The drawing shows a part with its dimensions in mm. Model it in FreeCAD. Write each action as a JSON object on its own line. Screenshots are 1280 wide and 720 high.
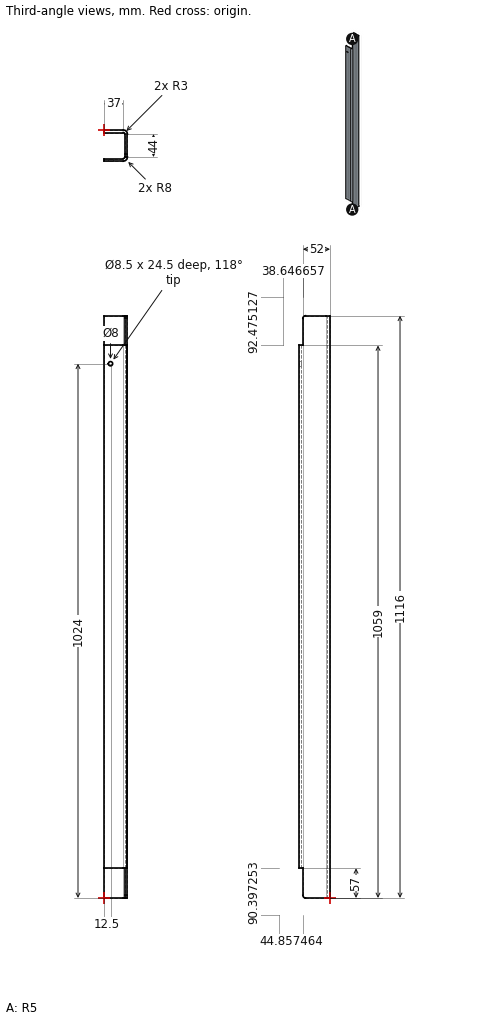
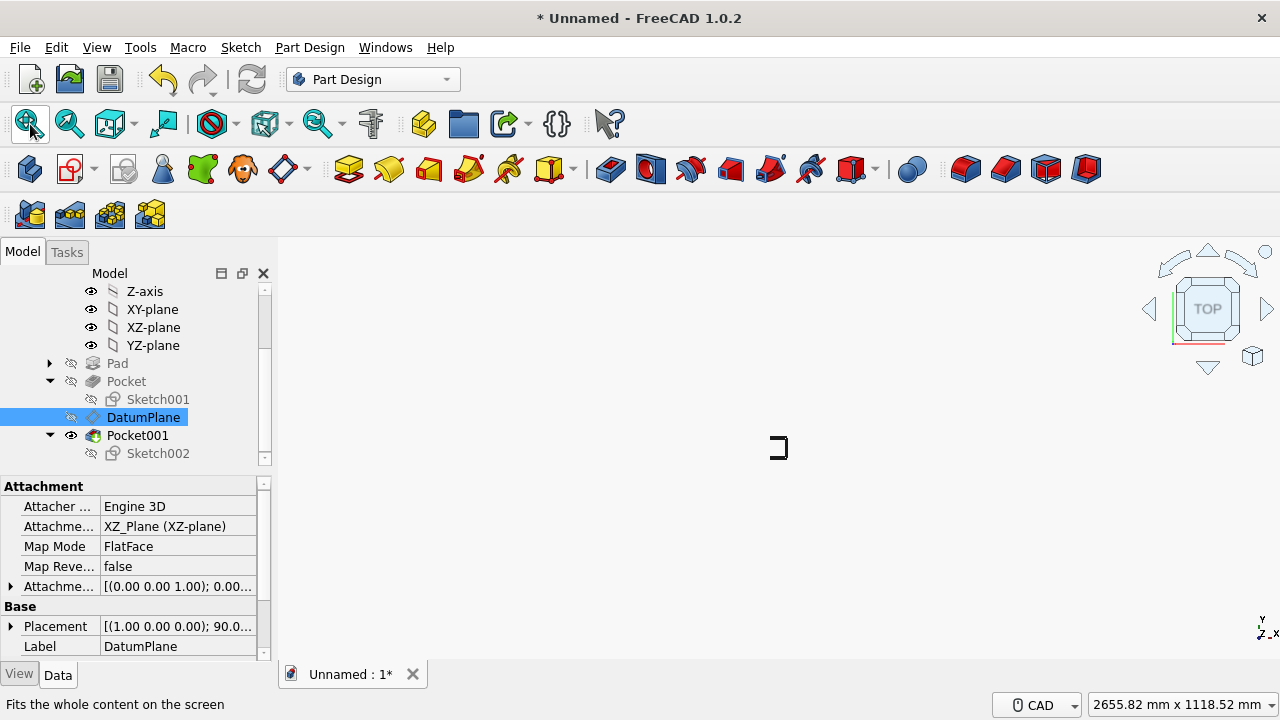
{"action": "scroll", "coordinate": [787, 455], "scroll_direction": "up", "scroll_amount": 15}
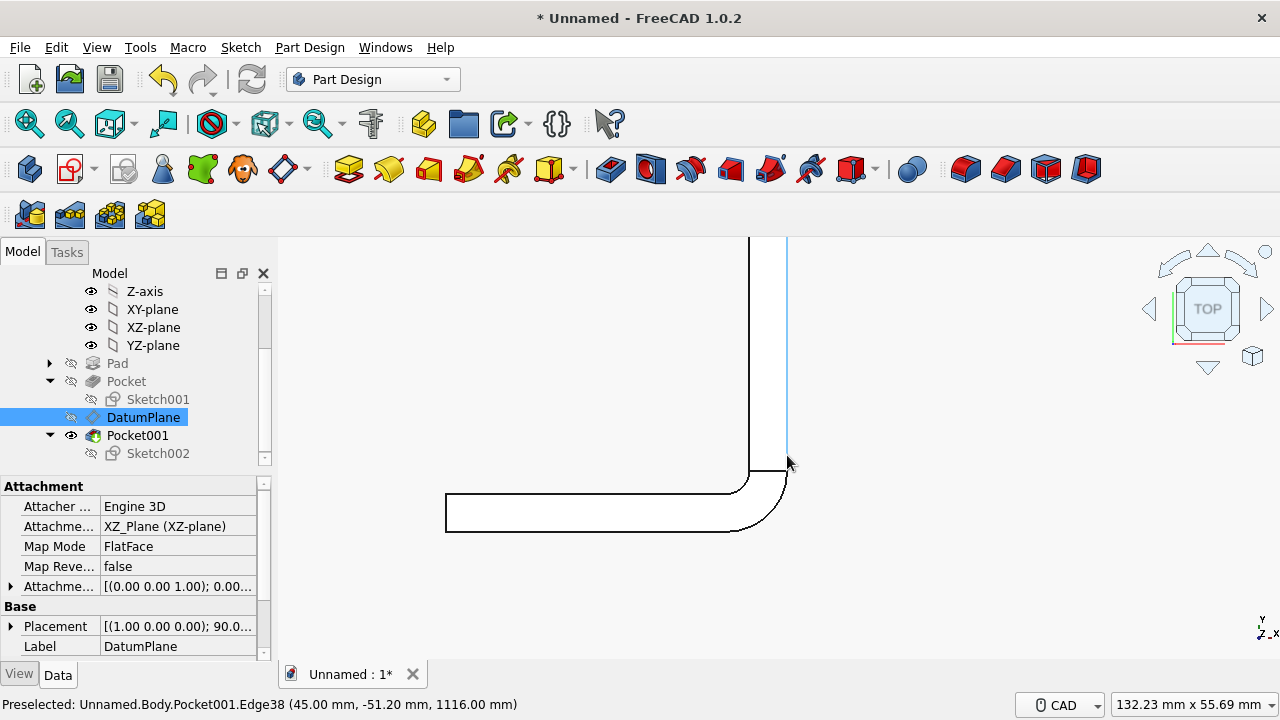
{"action": "left_click", "coordinate": [768, 470]}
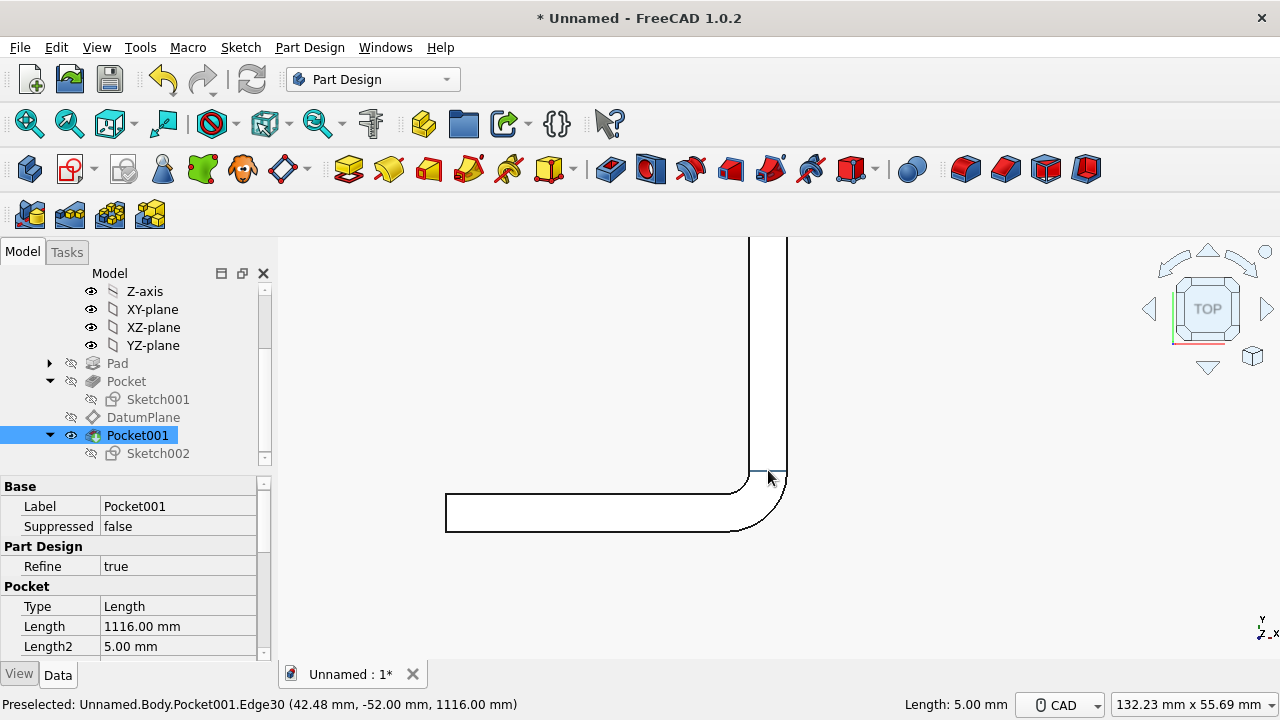
{"action": "key", "text": "v f"}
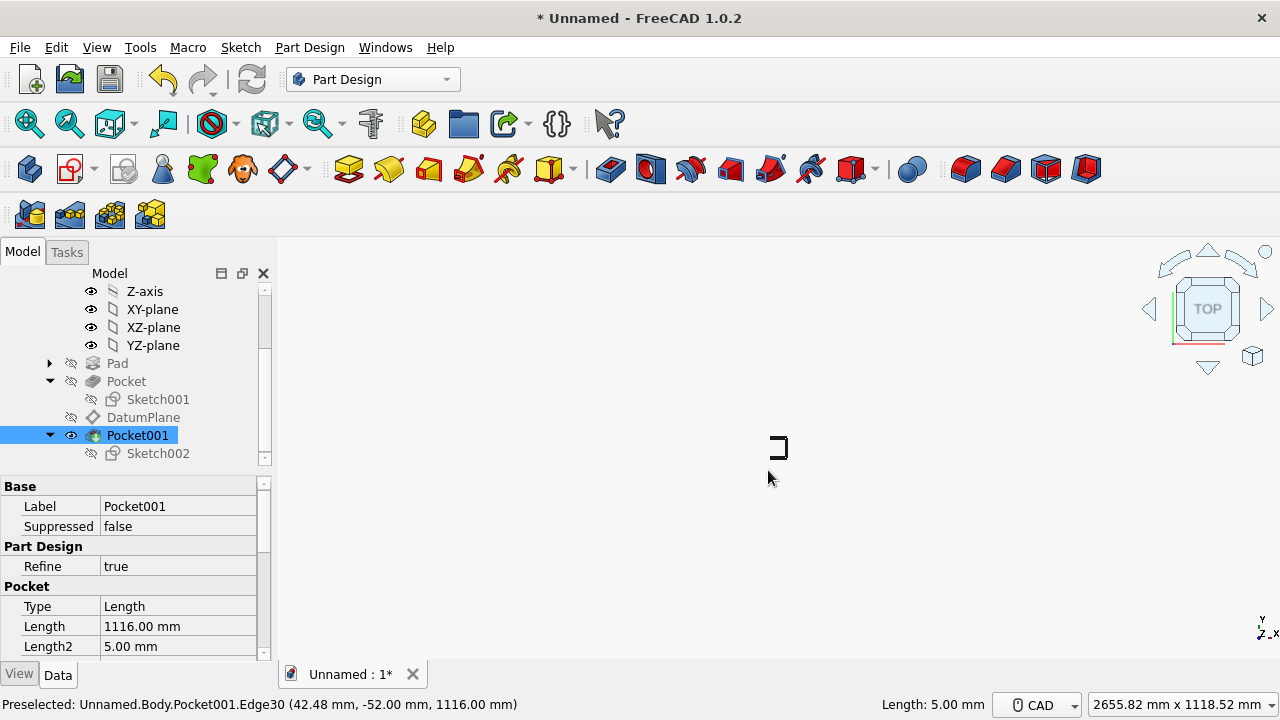
{"action": "key", "text": "1"}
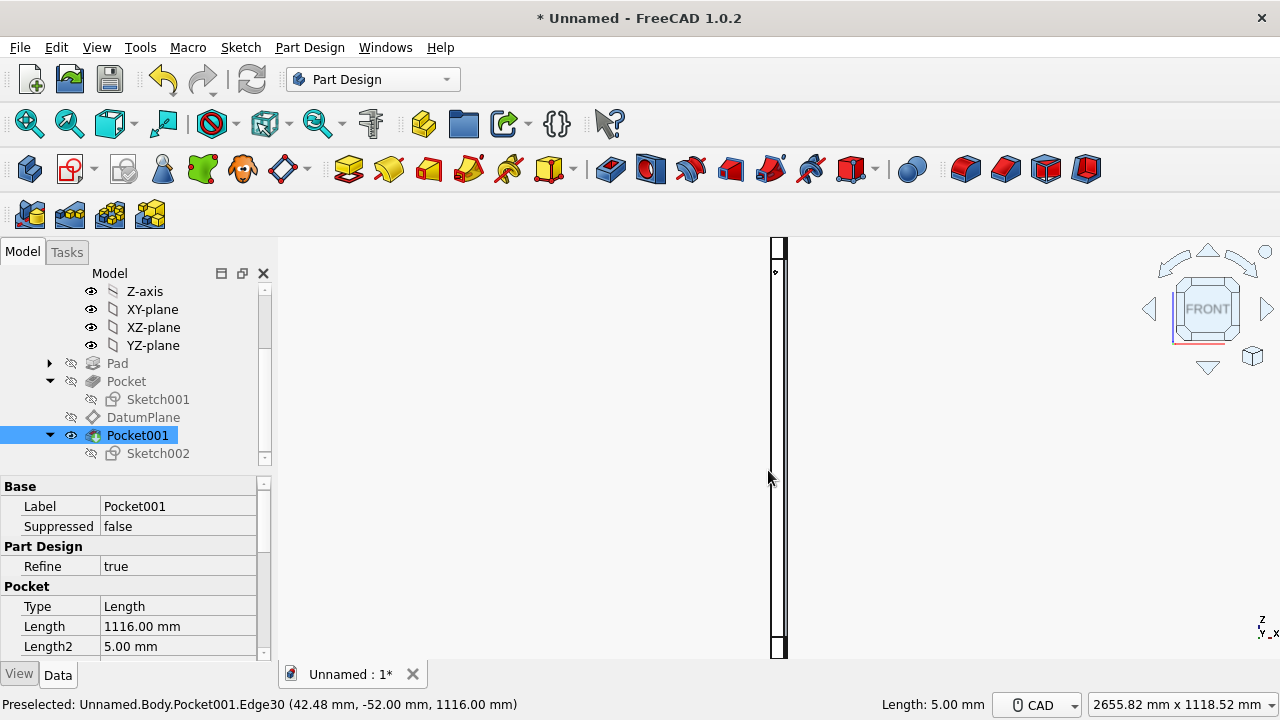
{"action": "left_click", "coordinate": [30, 124]}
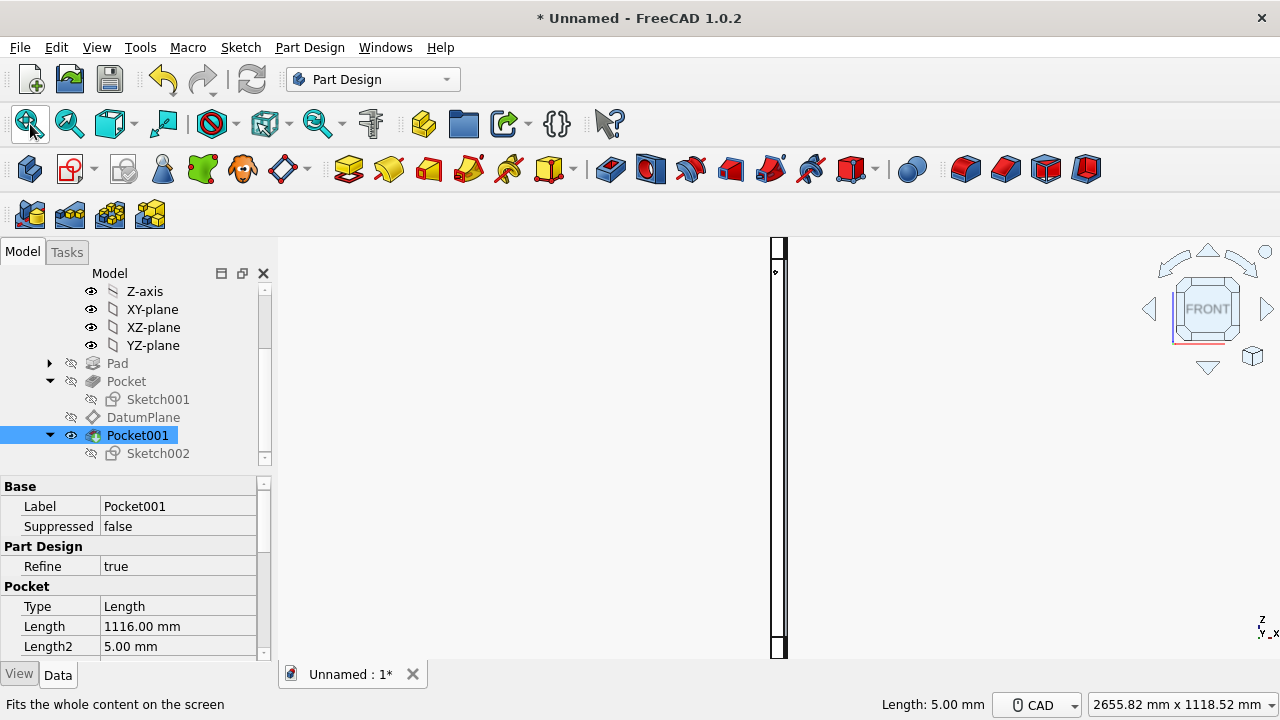
{"action": "key", "text": "3"}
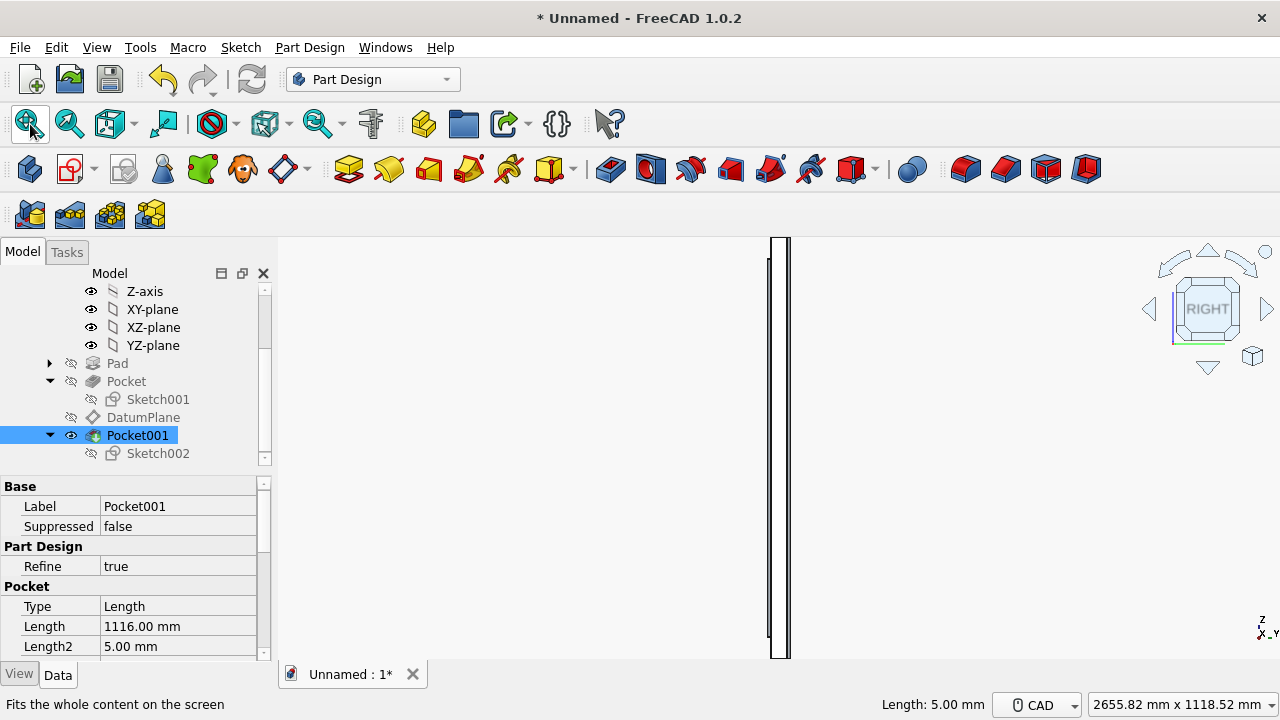
{"action": "key", "text": "v f"}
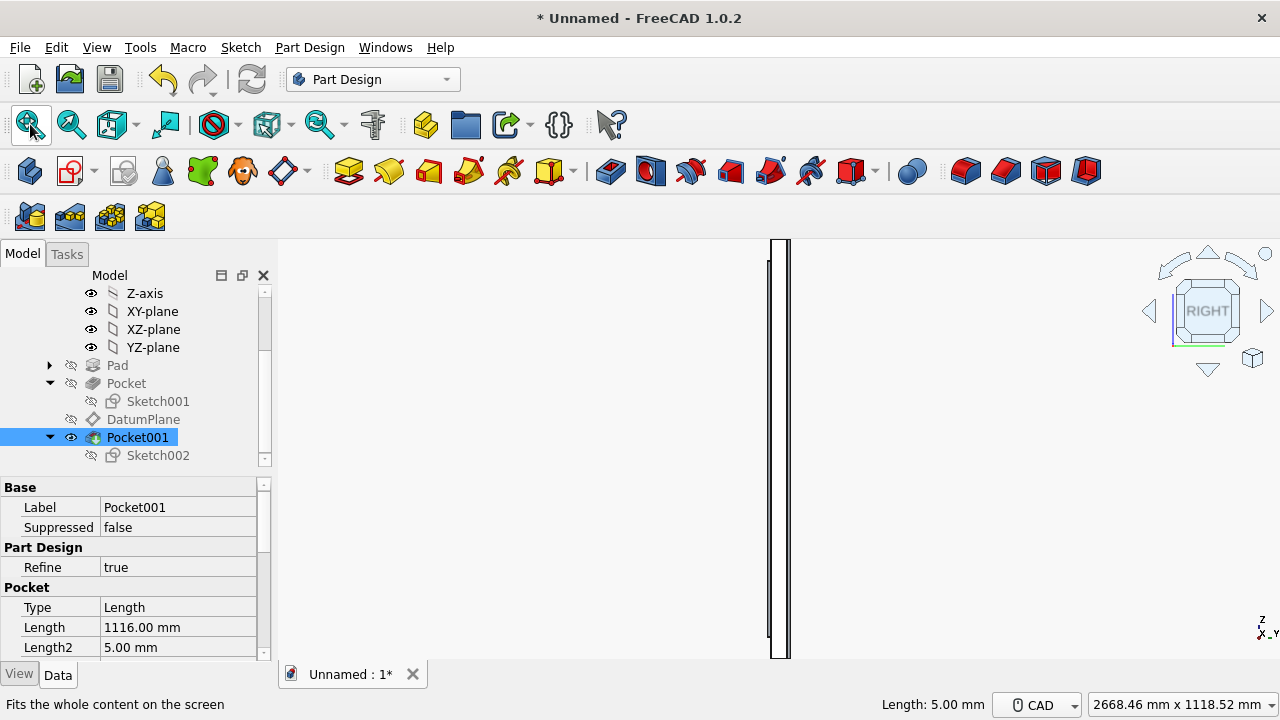
{"action": "key", "text": "5"}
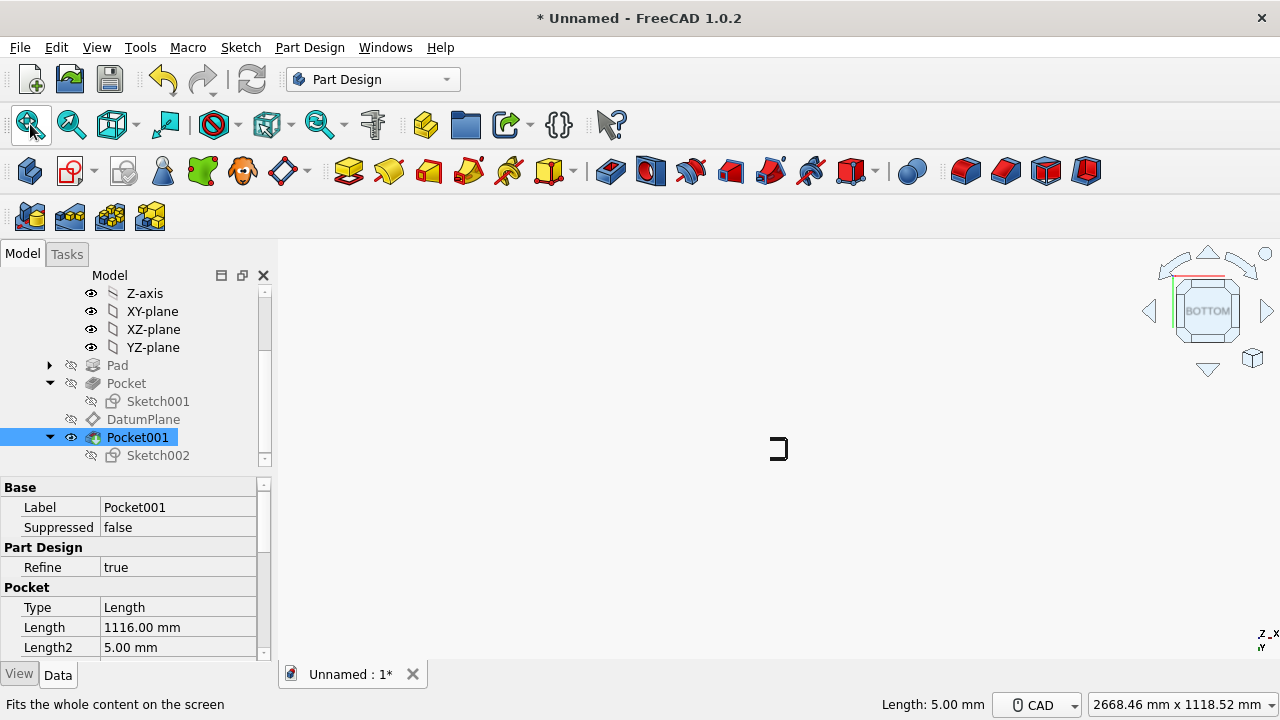
{"action": "key", "text": "v f"}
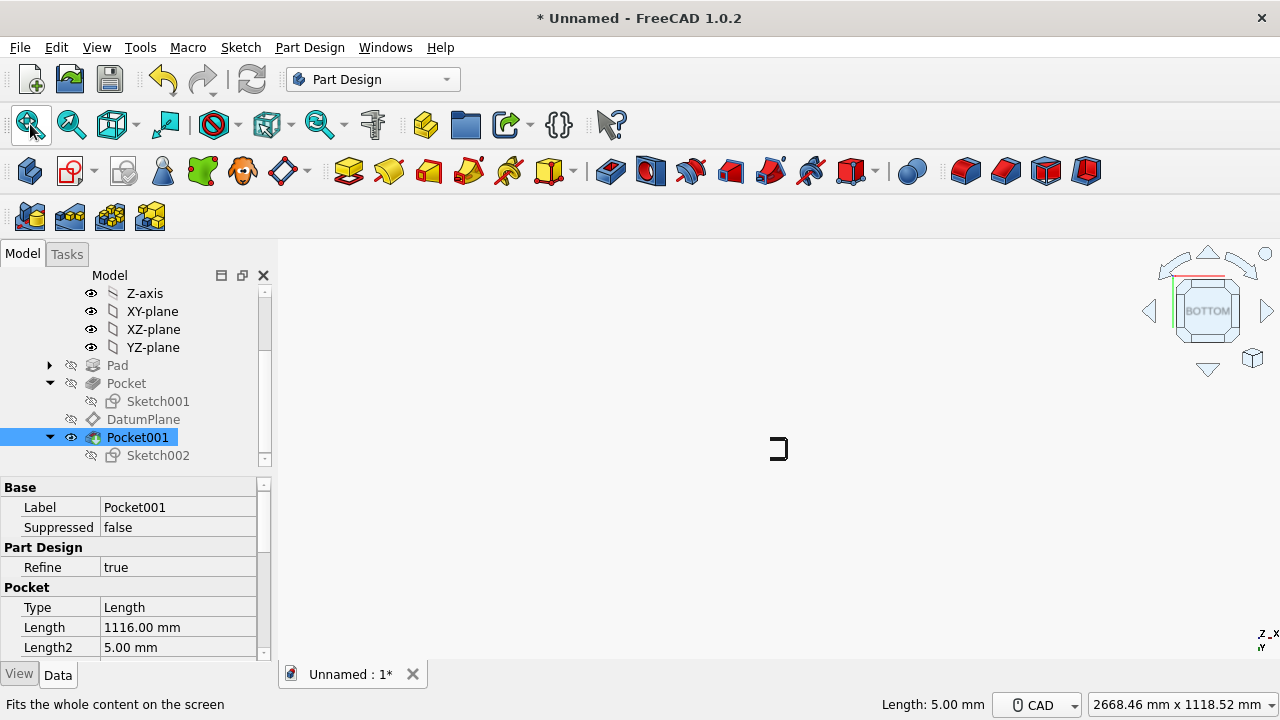
{"action": "scroll", "coordinate": [787, 440], "scroll_direction": "up", "scroll_amount": 15}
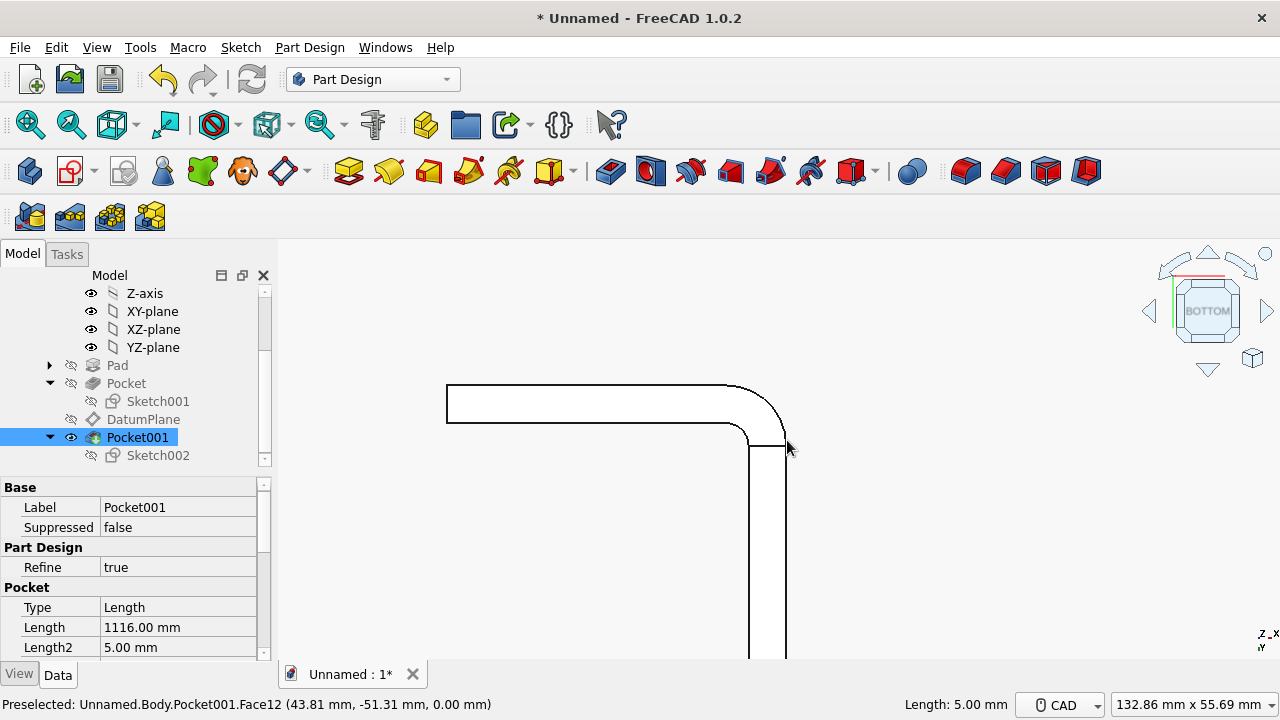
{"action": "left_click", "coordinate": [767, 445], "text": "ctrl"}